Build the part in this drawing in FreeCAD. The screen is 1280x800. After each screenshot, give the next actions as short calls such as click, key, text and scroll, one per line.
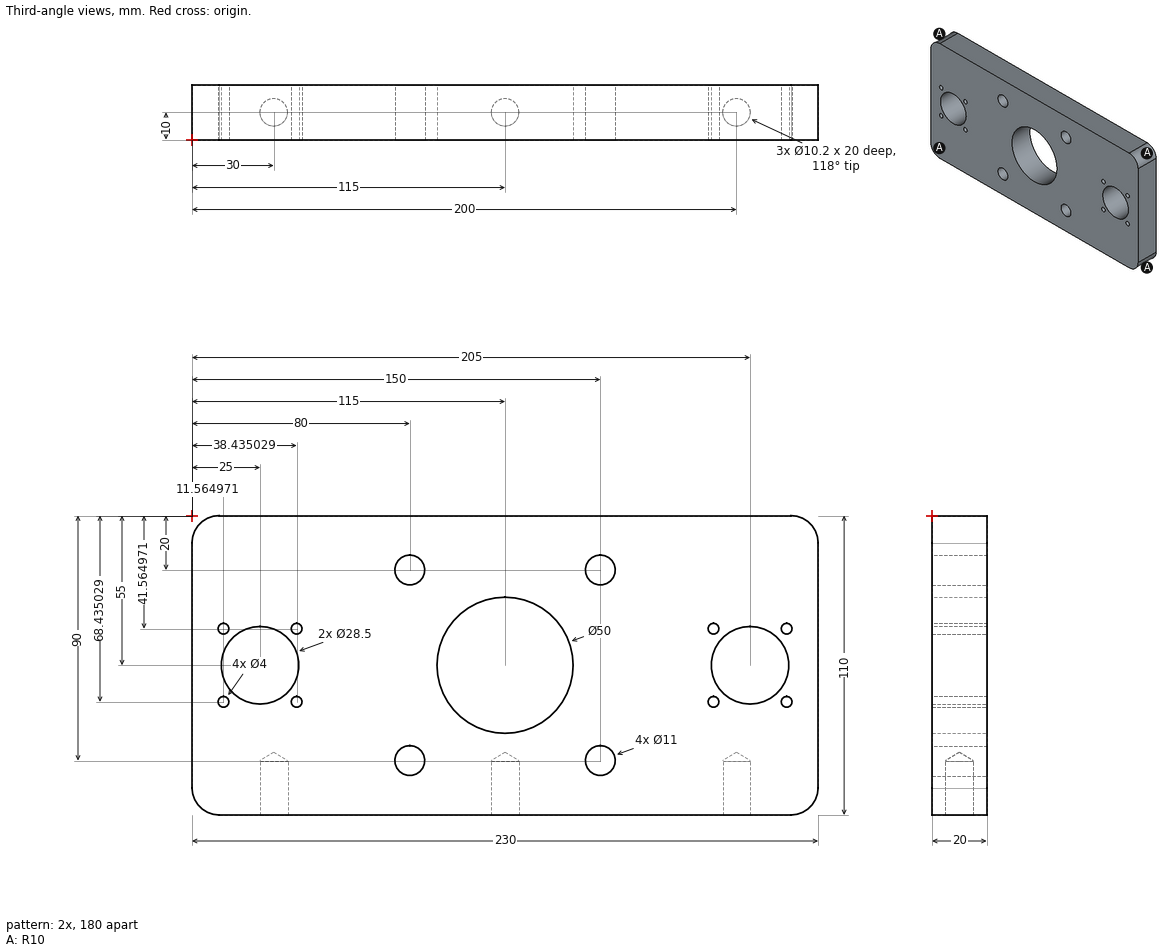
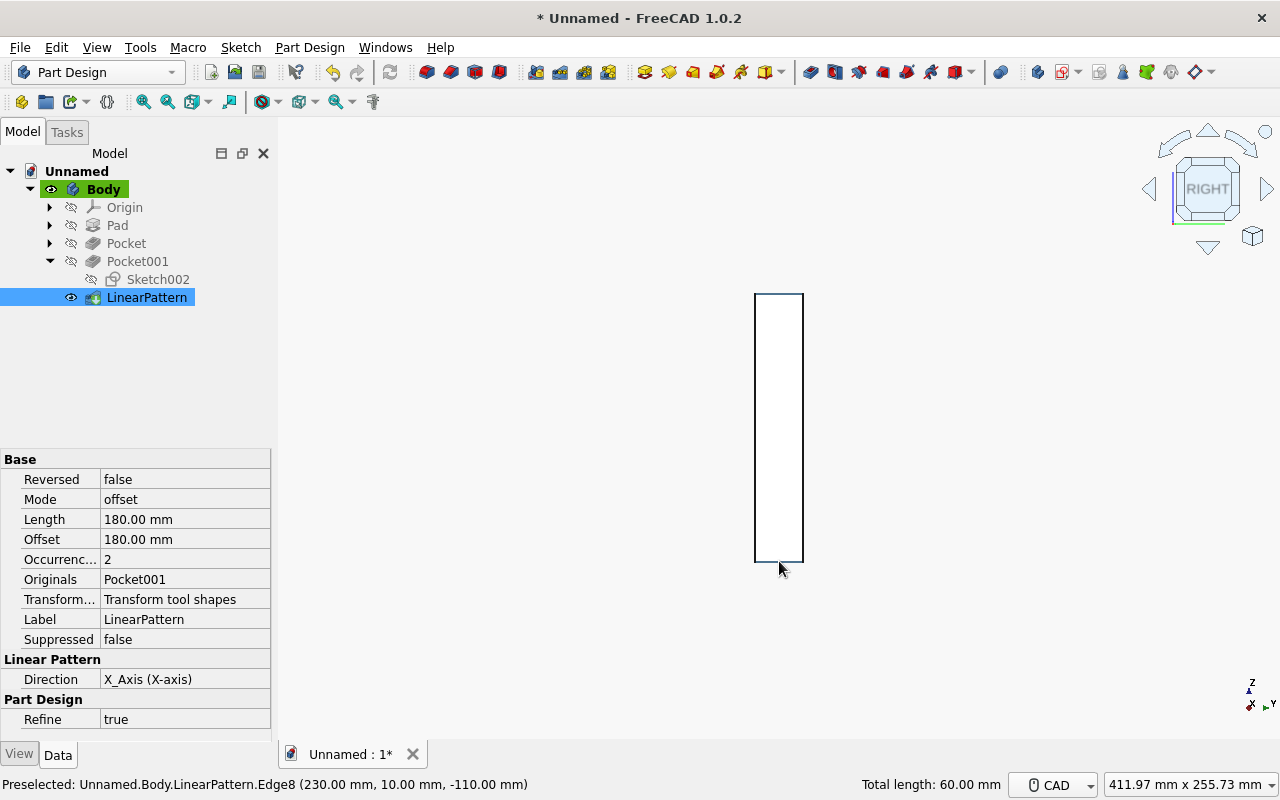
key(5)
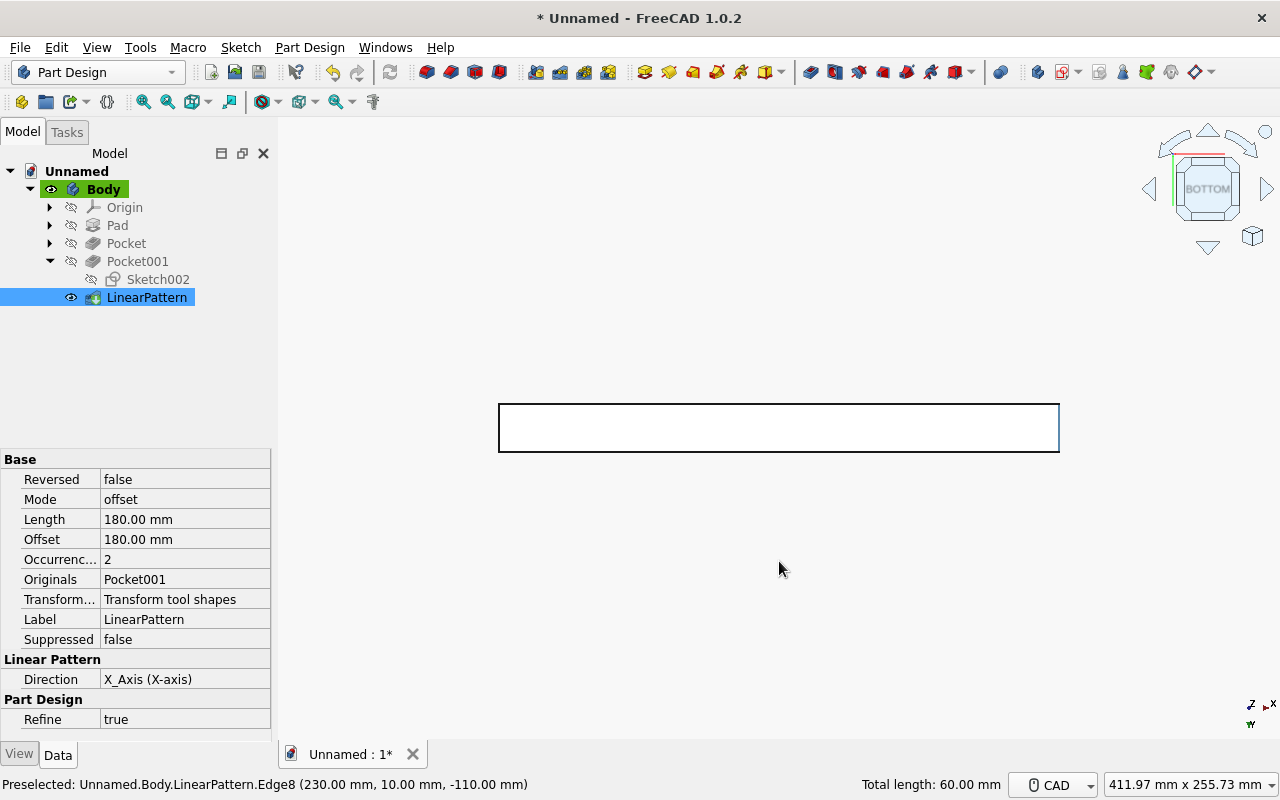
click(499, 427, ctrl)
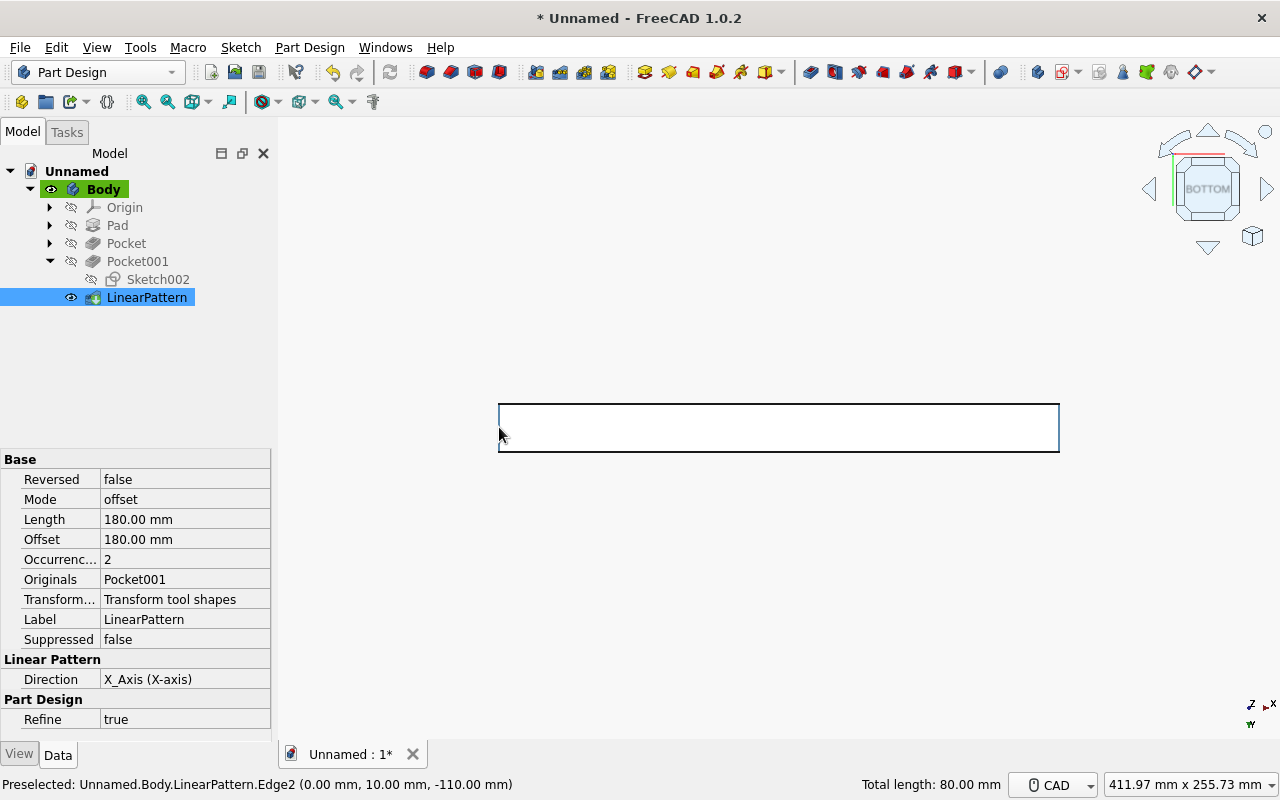
click(428, 72)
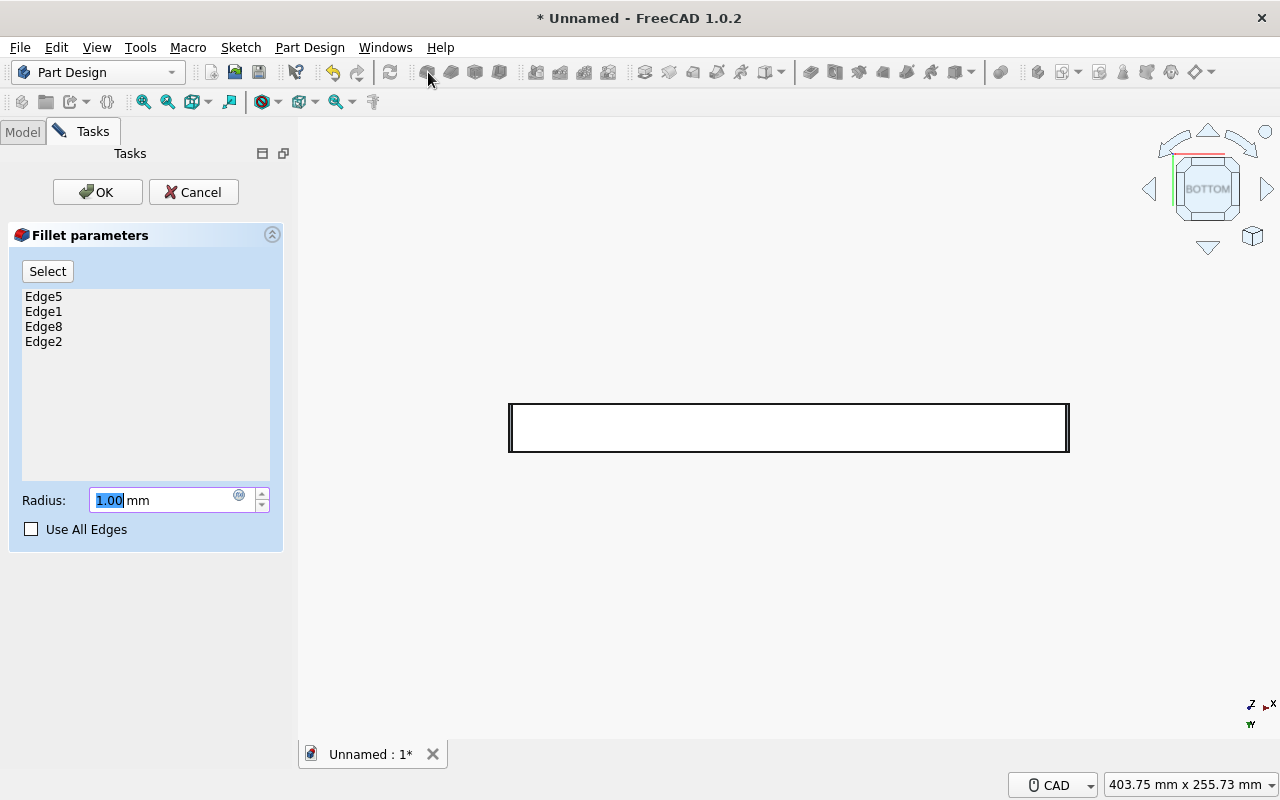
text(10)
key(Tab)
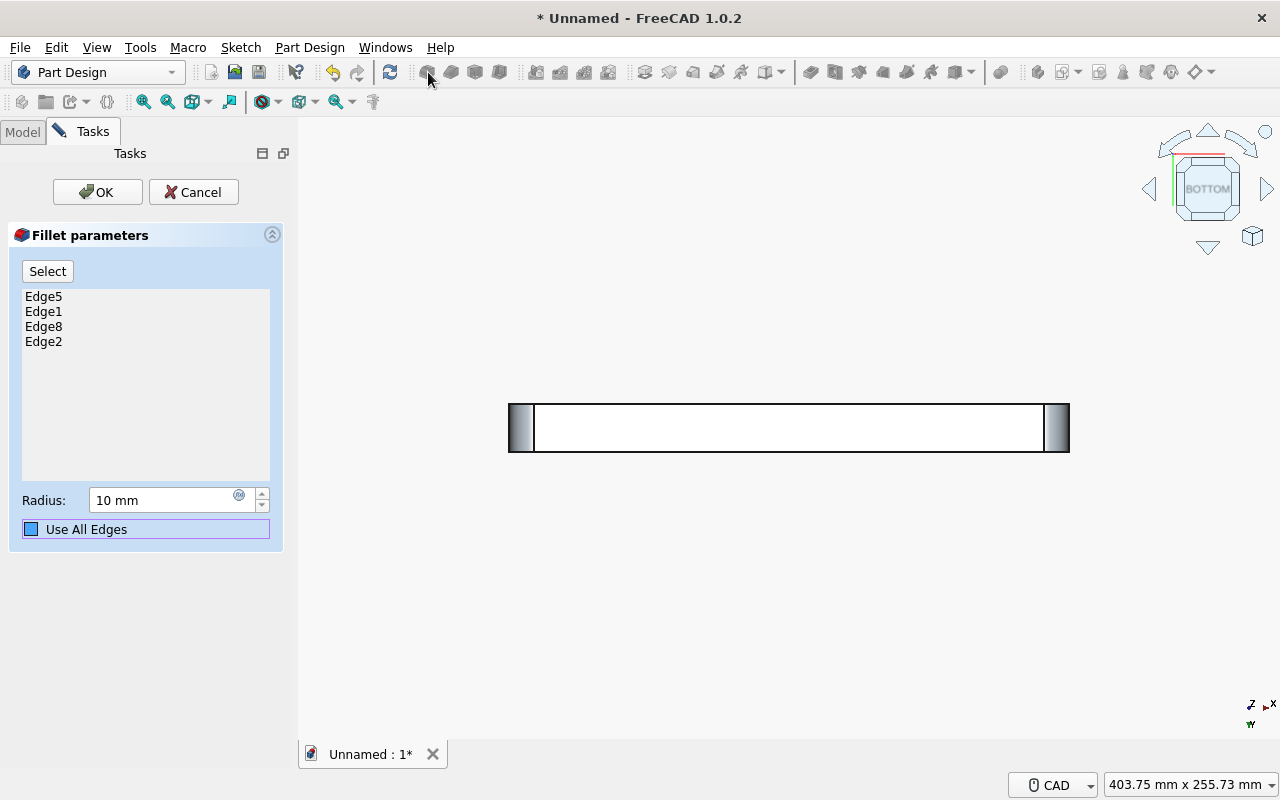
click(98, 192)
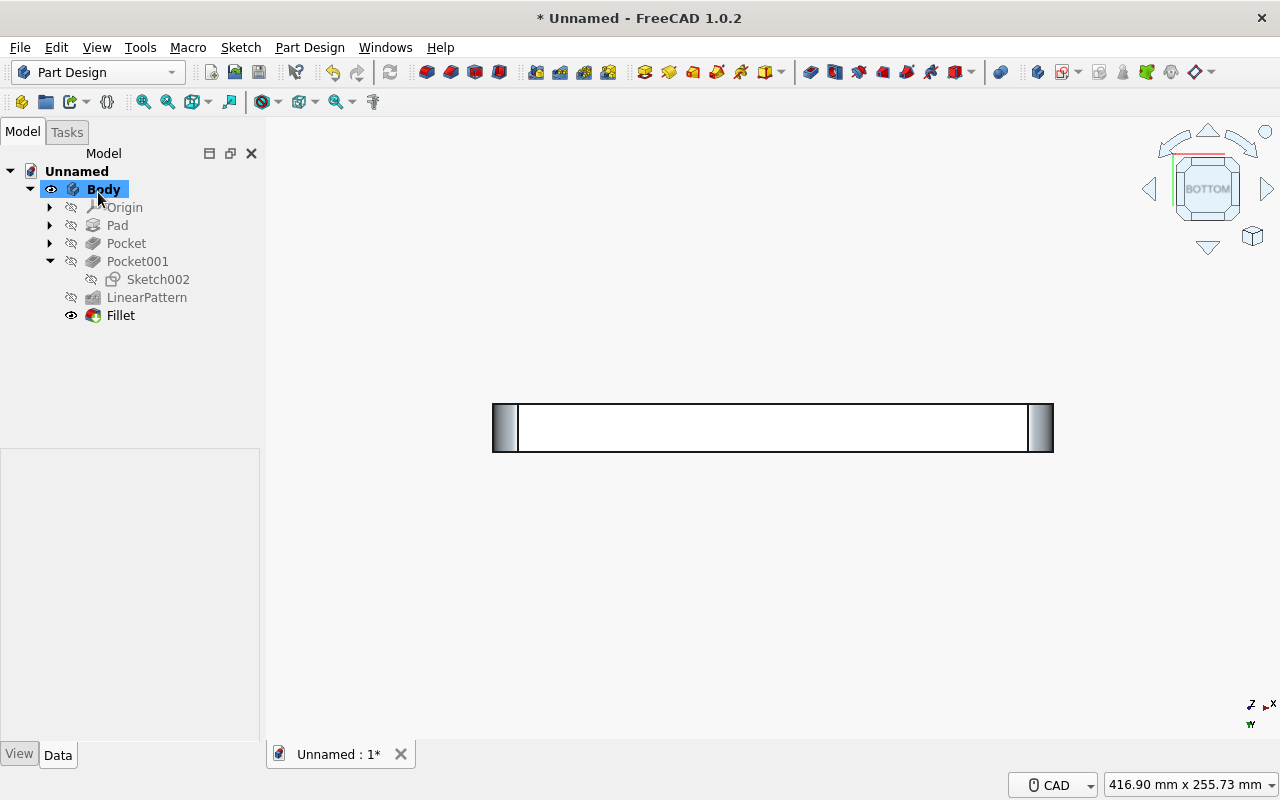
key(4)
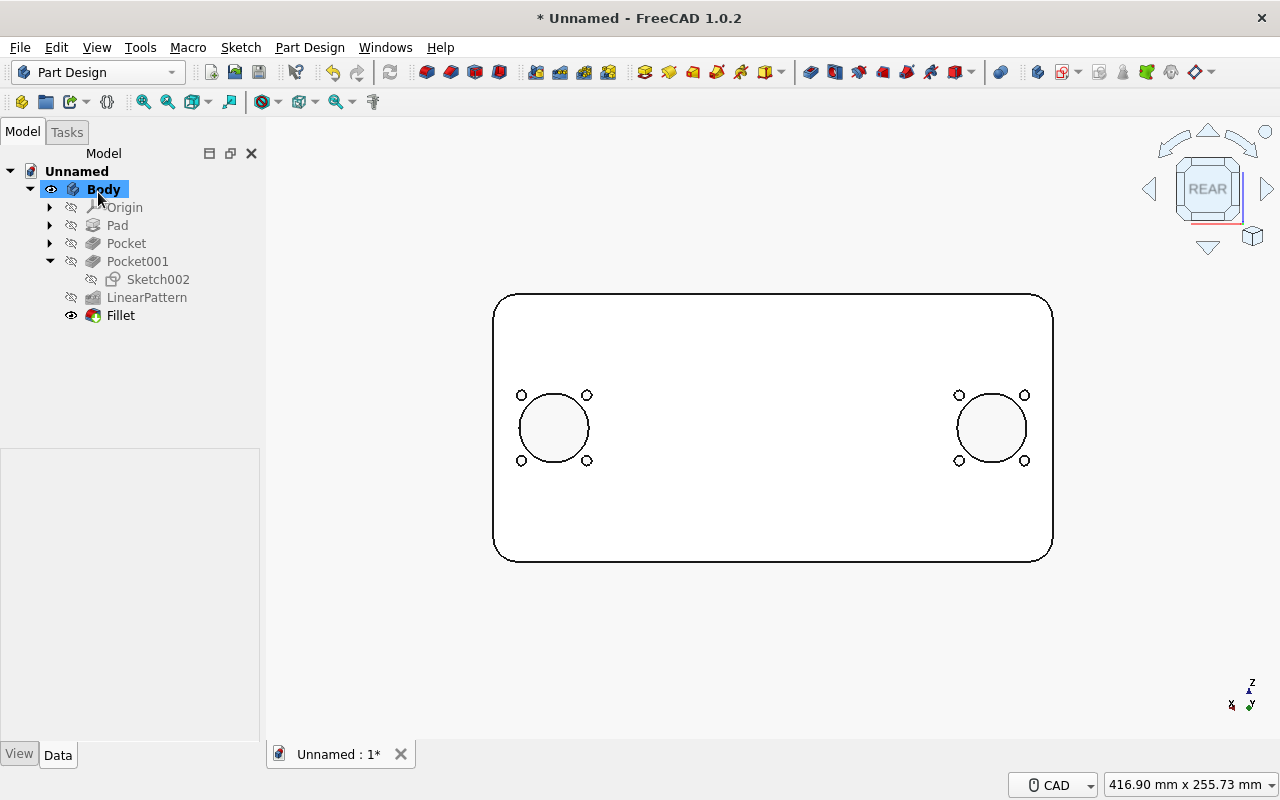
click(773, 427)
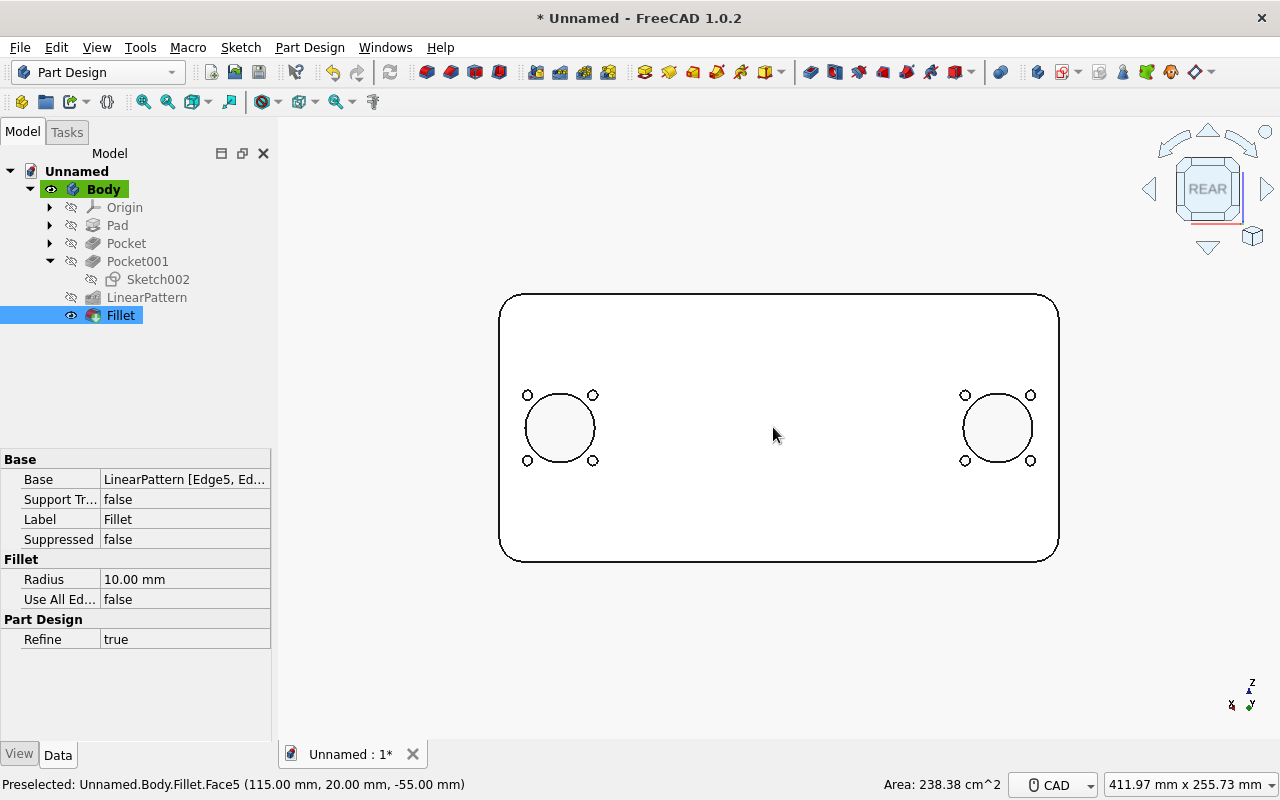
click(1062, 72)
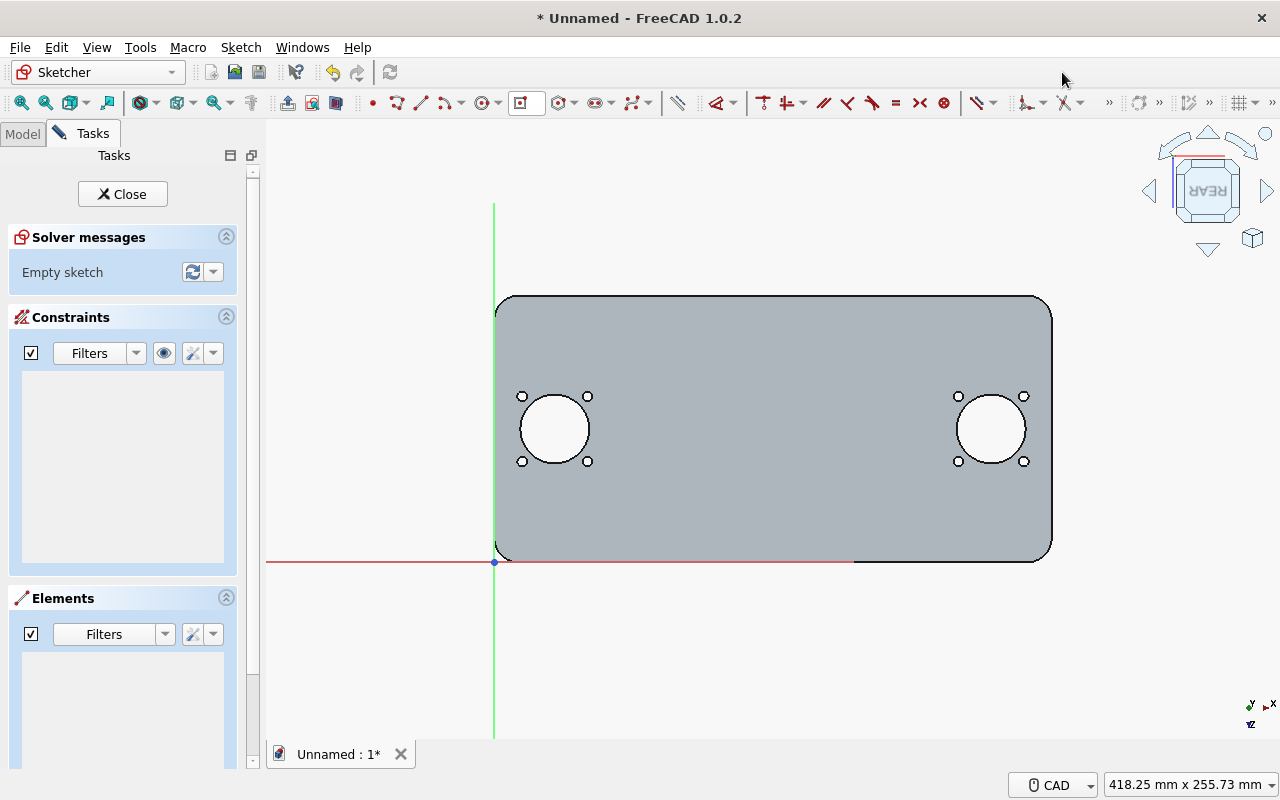
scroll(638, 482, up, 2)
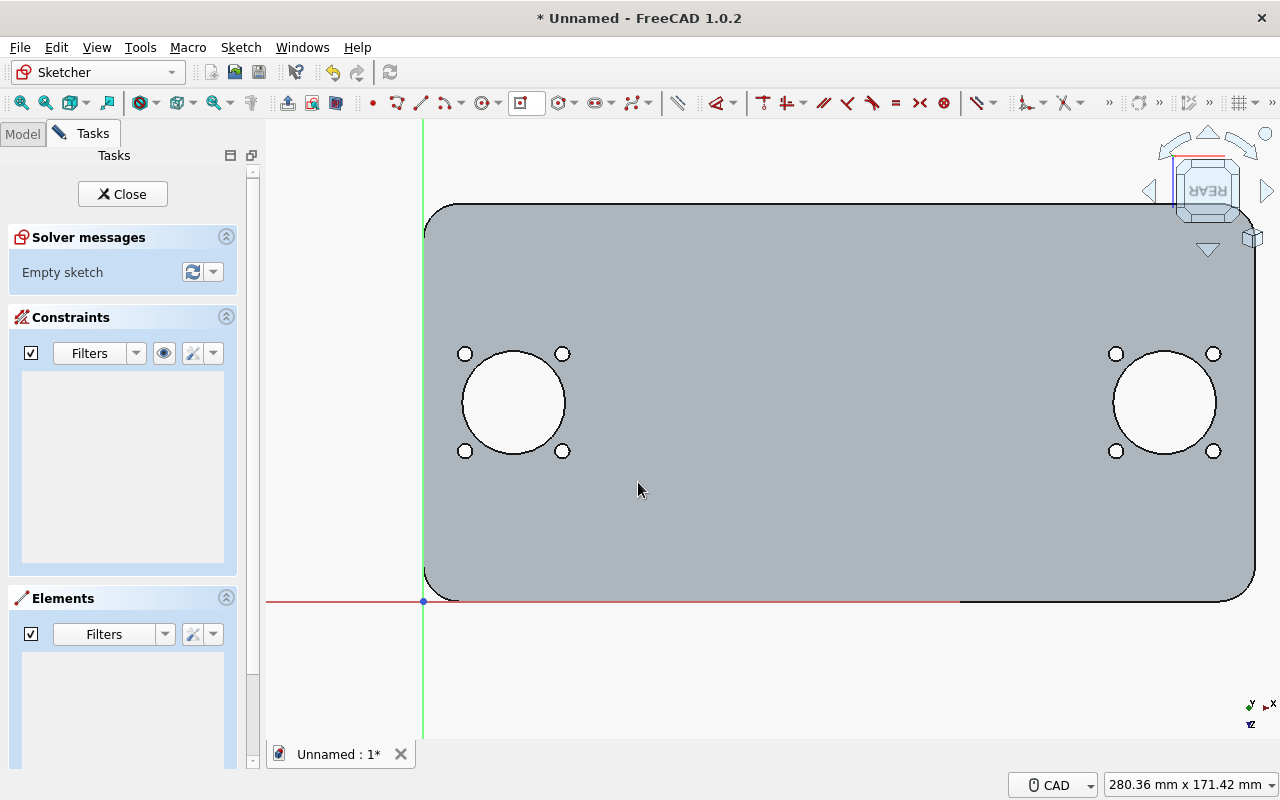
key(g)
key(c)